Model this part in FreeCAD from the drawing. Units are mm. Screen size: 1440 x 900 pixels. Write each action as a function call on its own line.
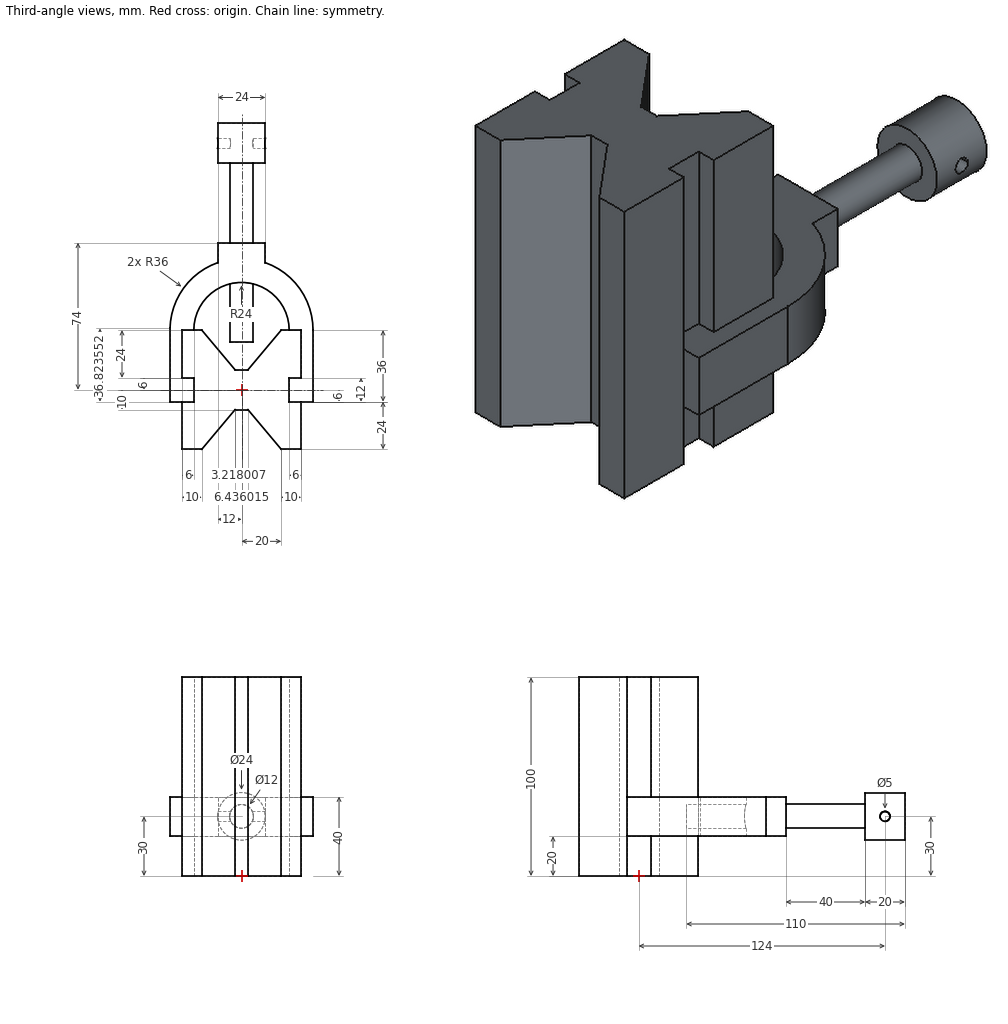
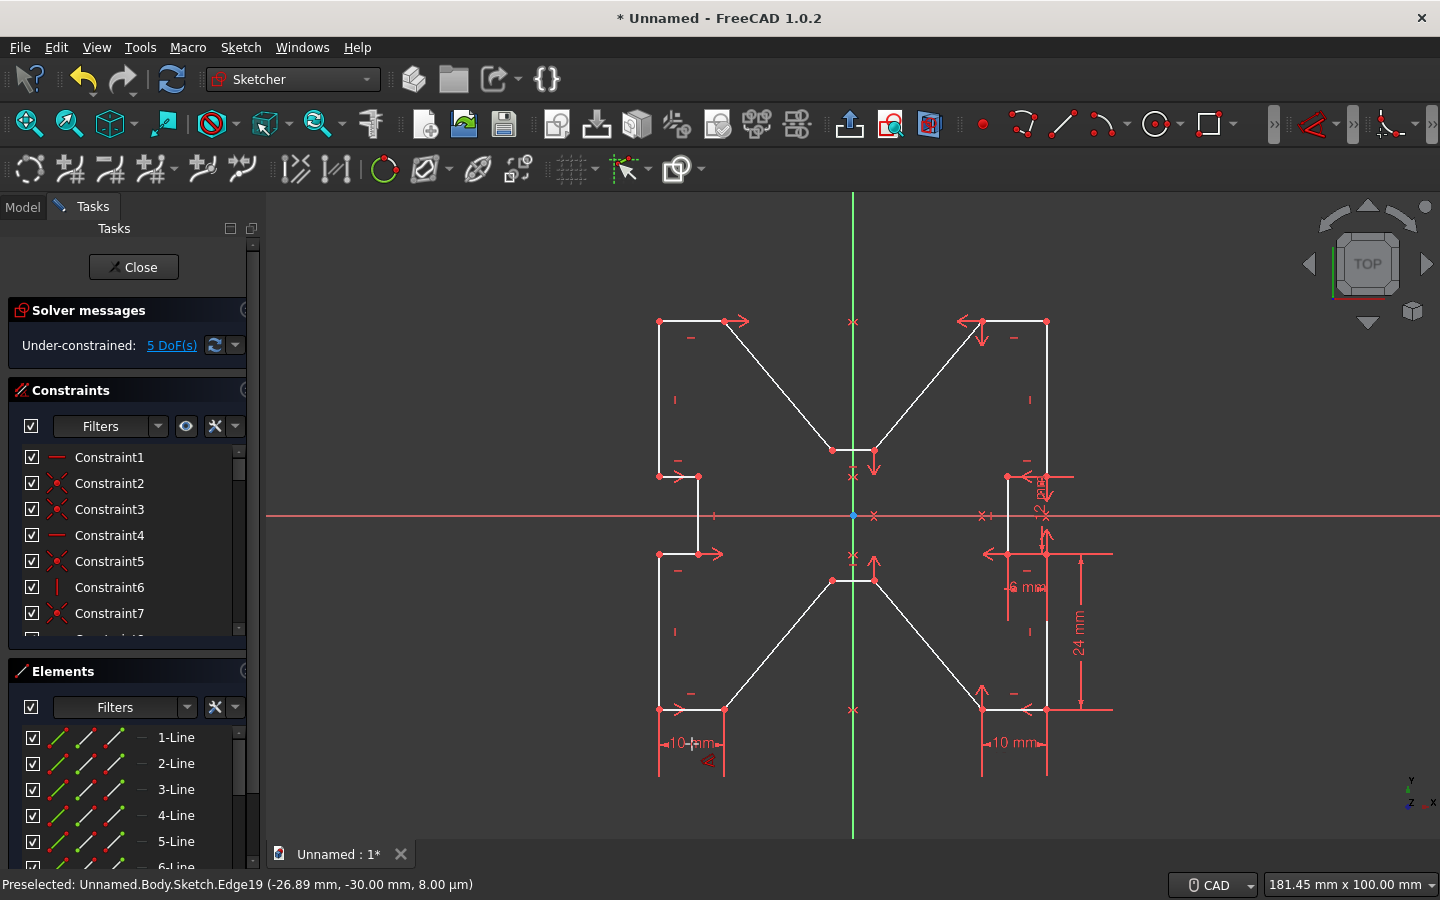
click(832, 581)
click(798, 548)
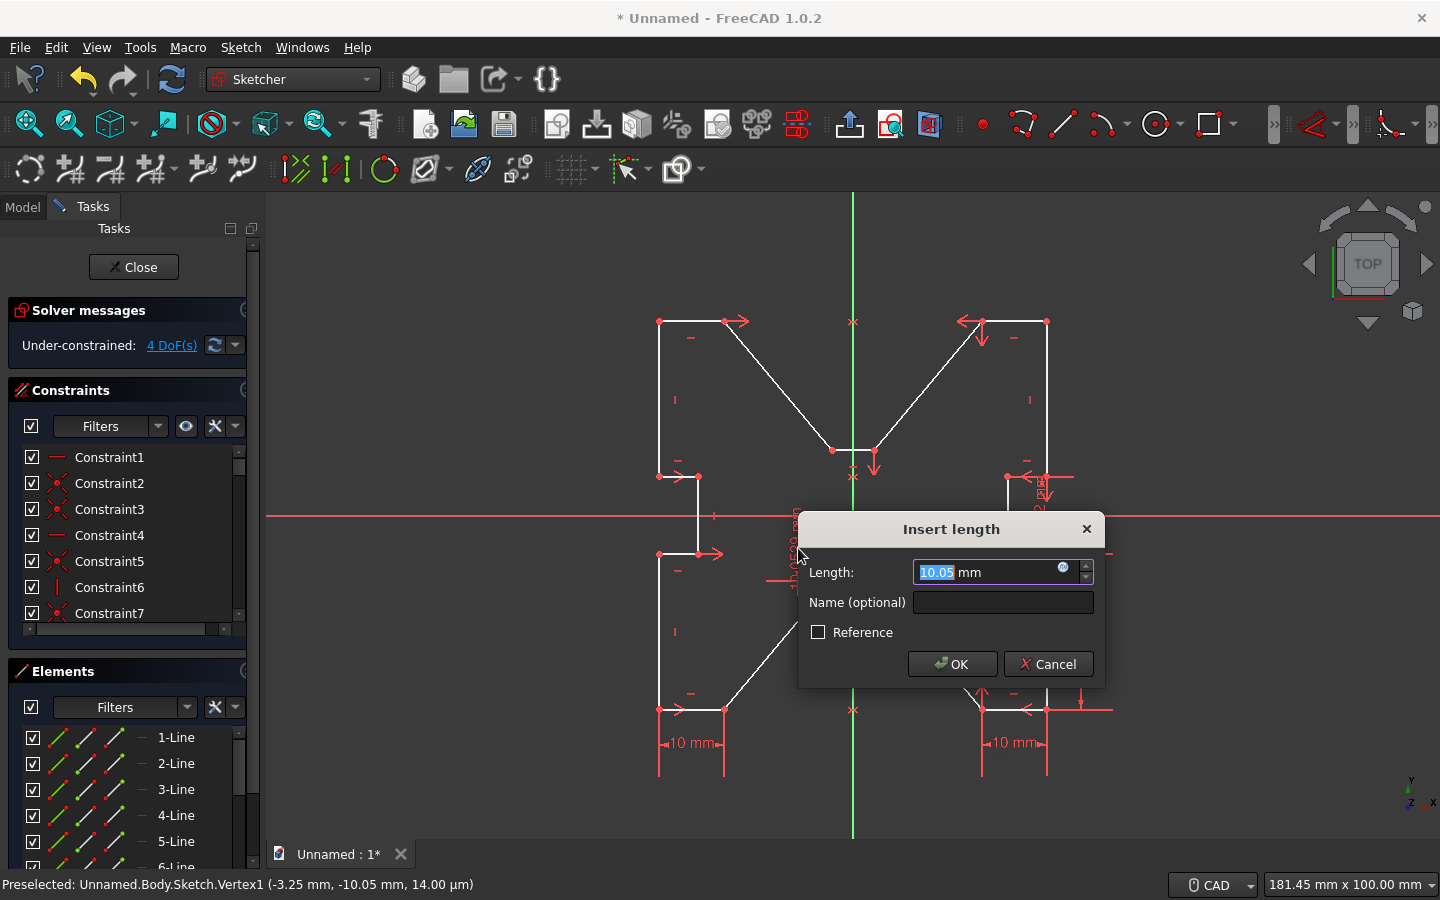
text(10)
key(Return)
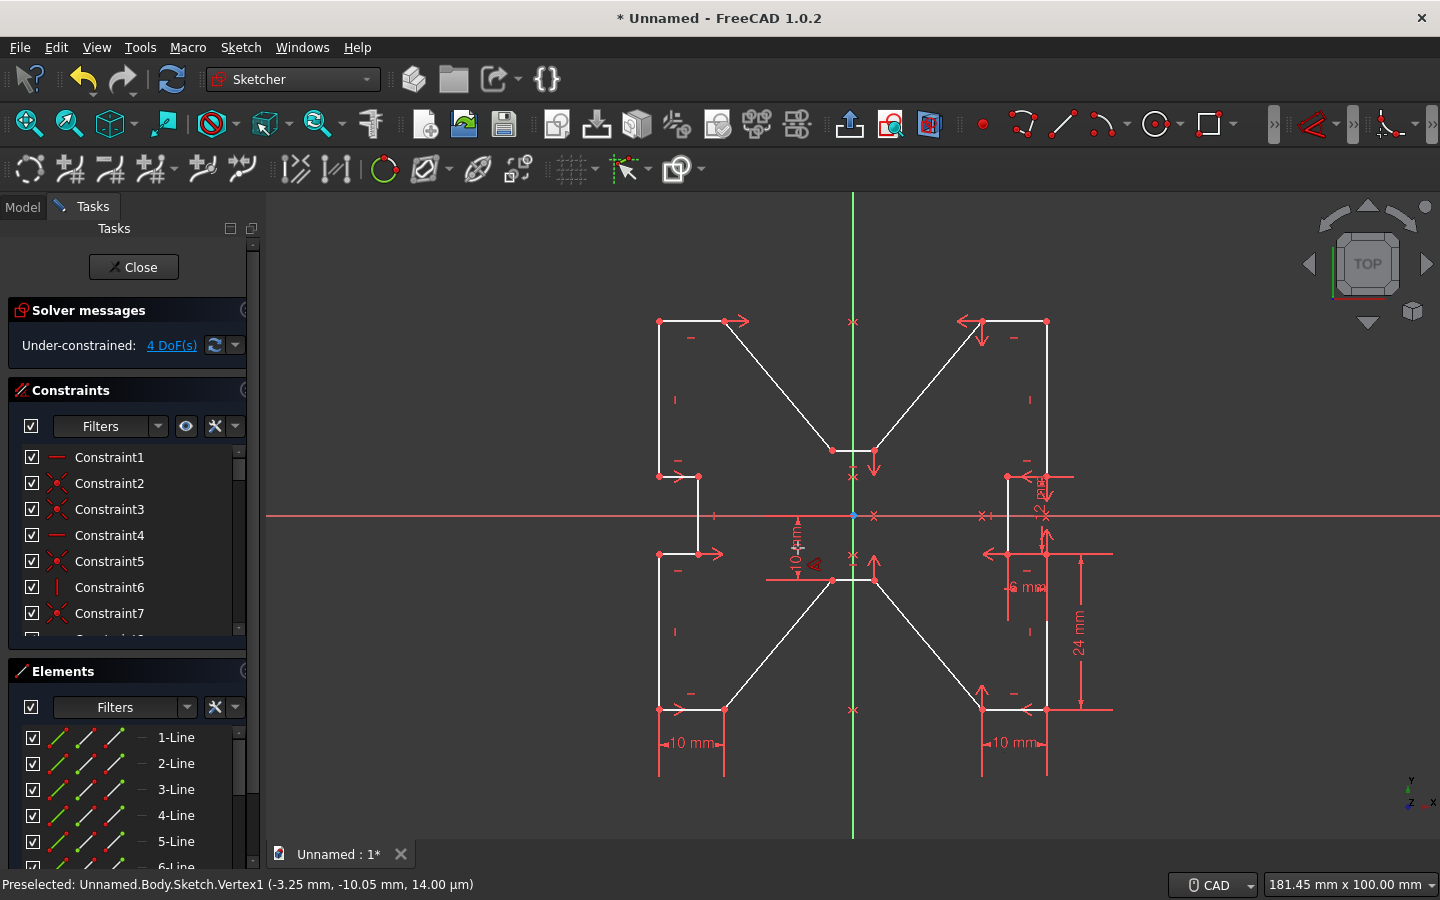
click(982, 710)
click(918, 744)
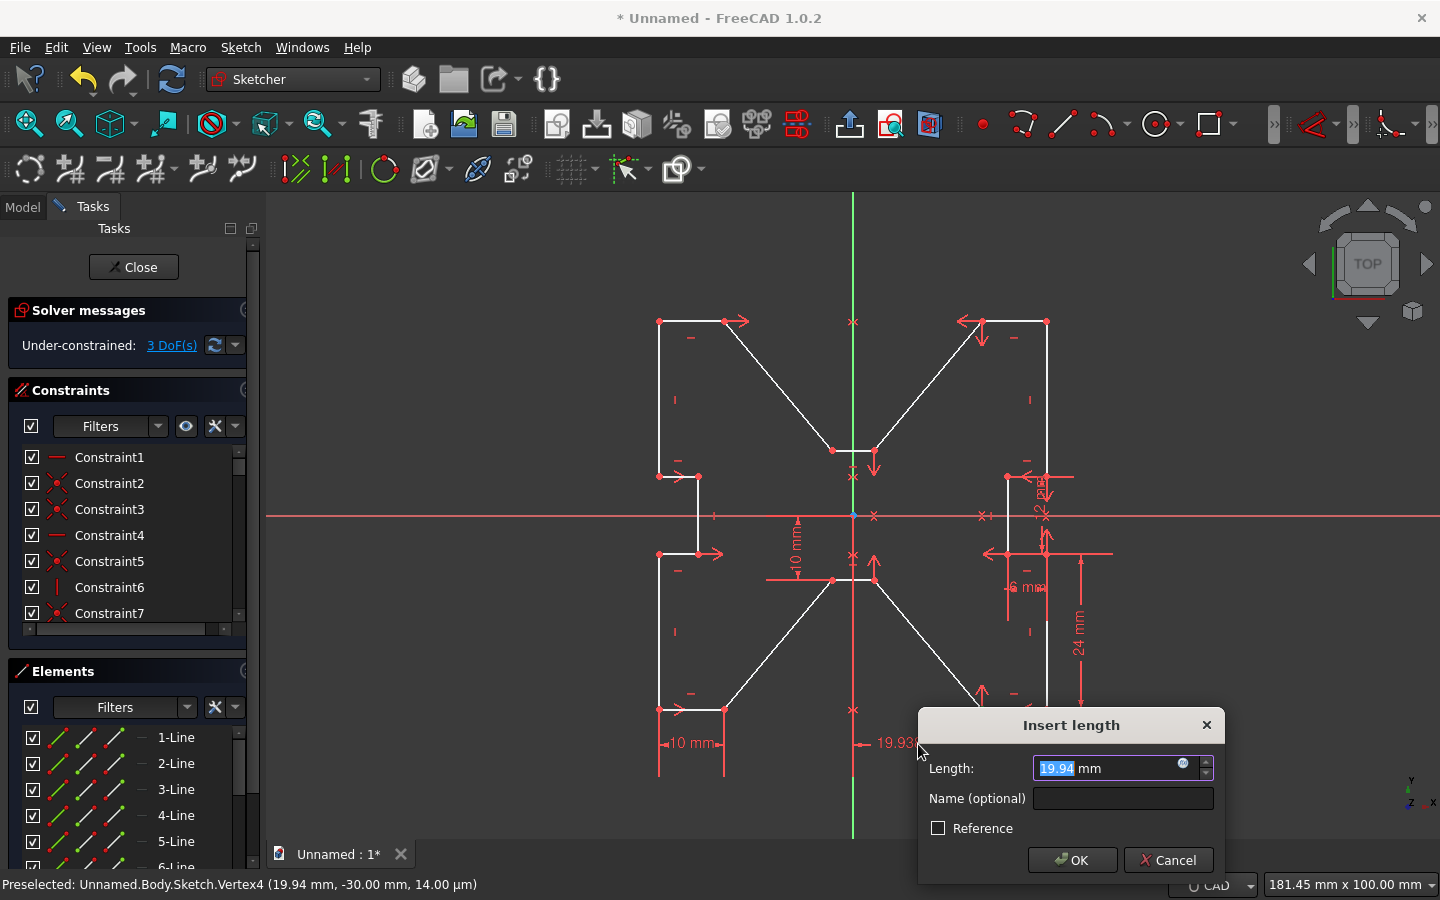
text(20)
key(Return)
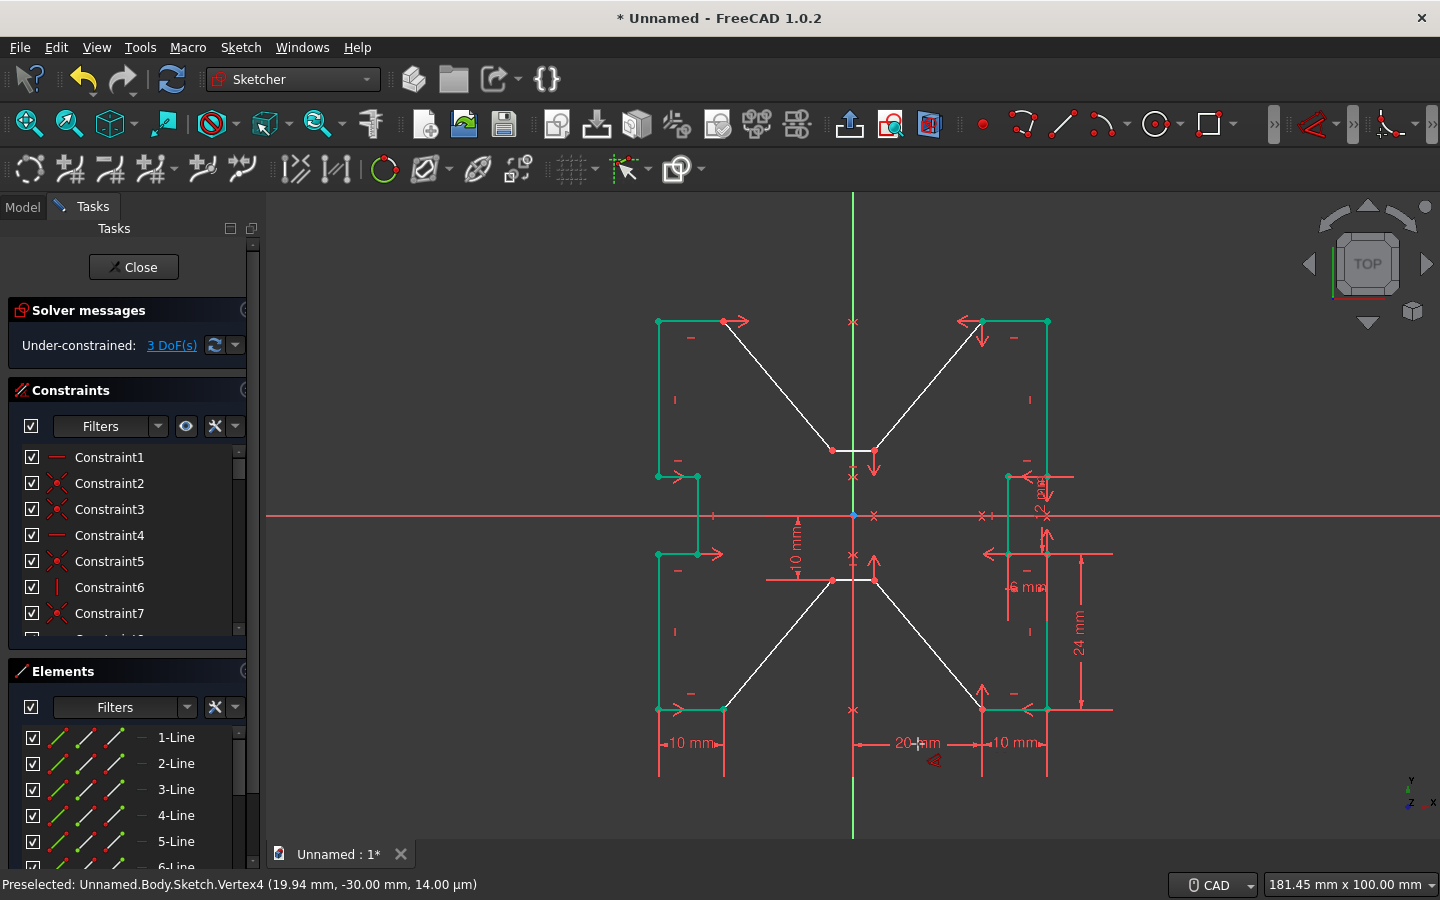
click(853, 580)
click(838, 614)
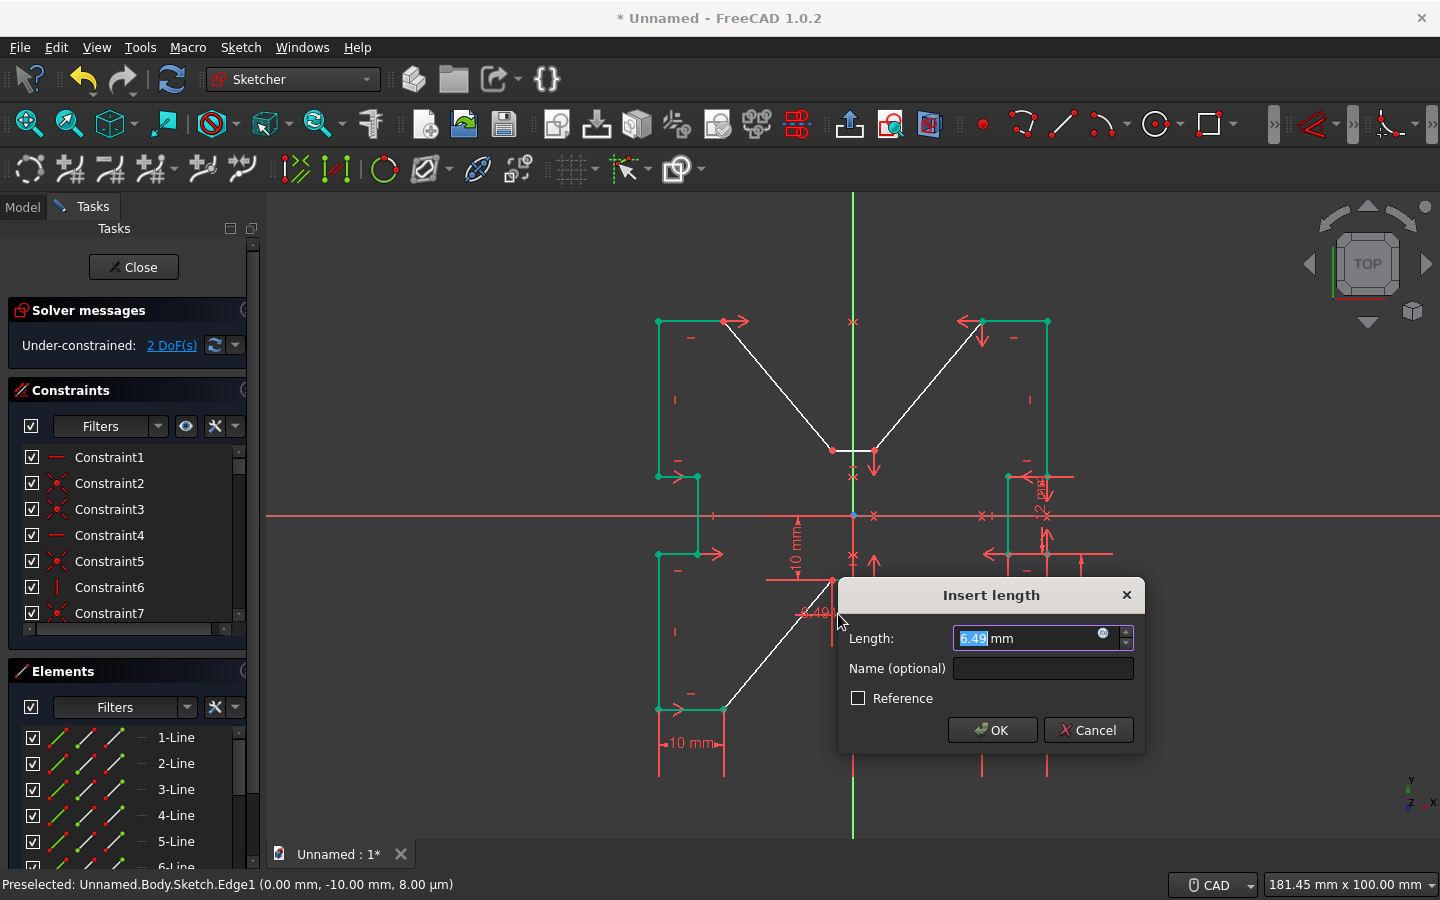
text(6.436015)
key(Return)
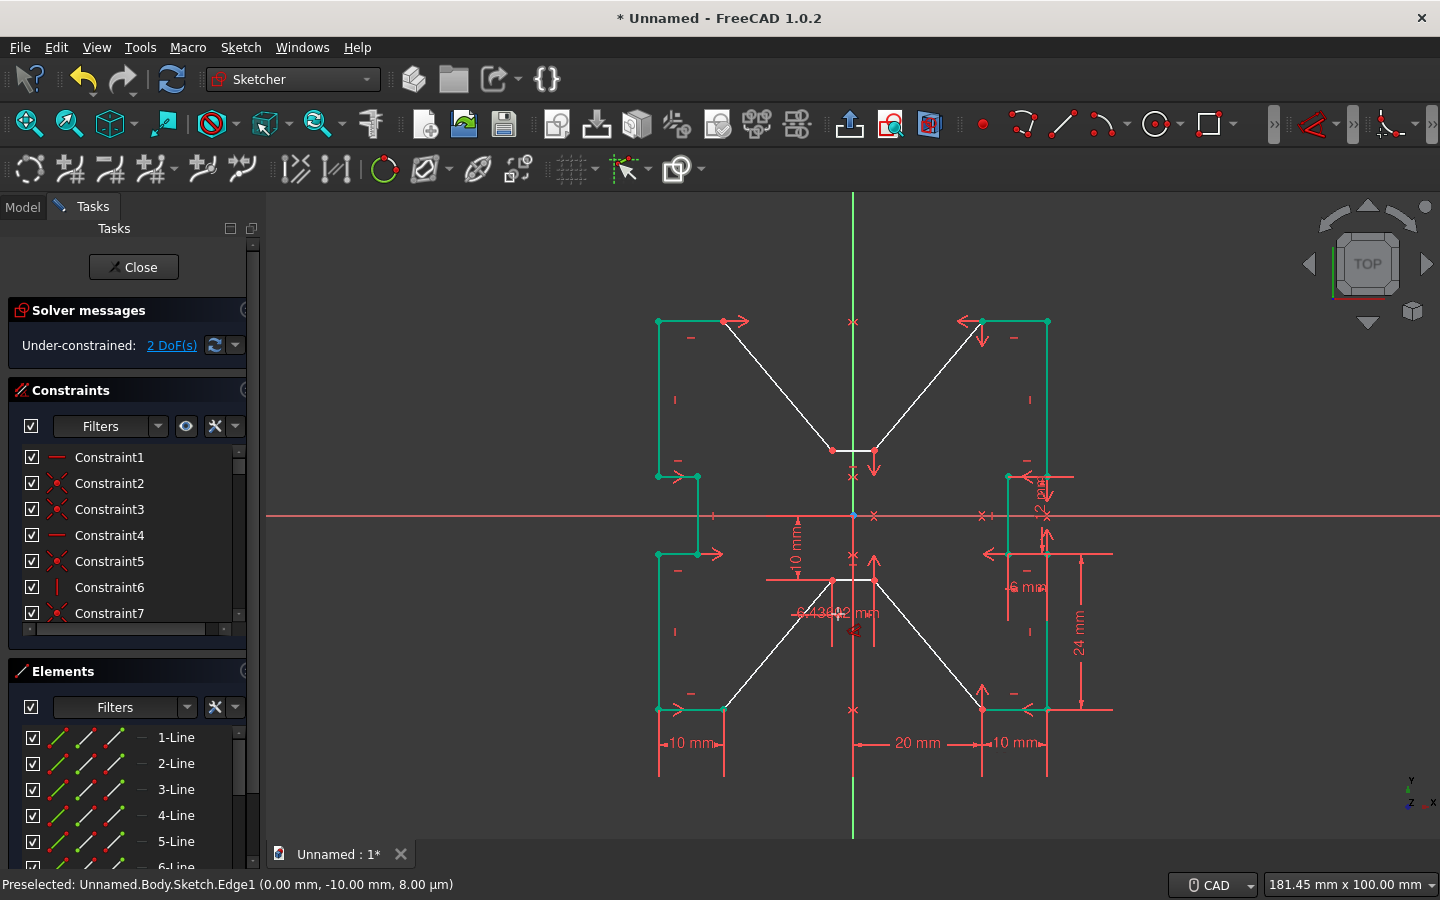
click(853, 451)
click(838, 417)